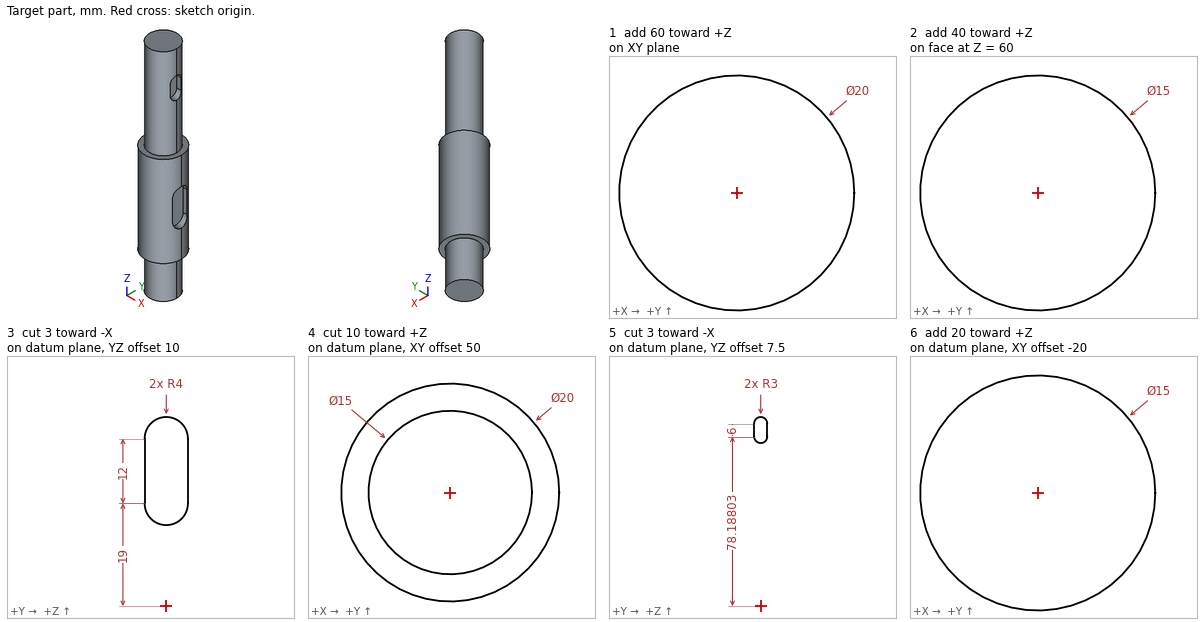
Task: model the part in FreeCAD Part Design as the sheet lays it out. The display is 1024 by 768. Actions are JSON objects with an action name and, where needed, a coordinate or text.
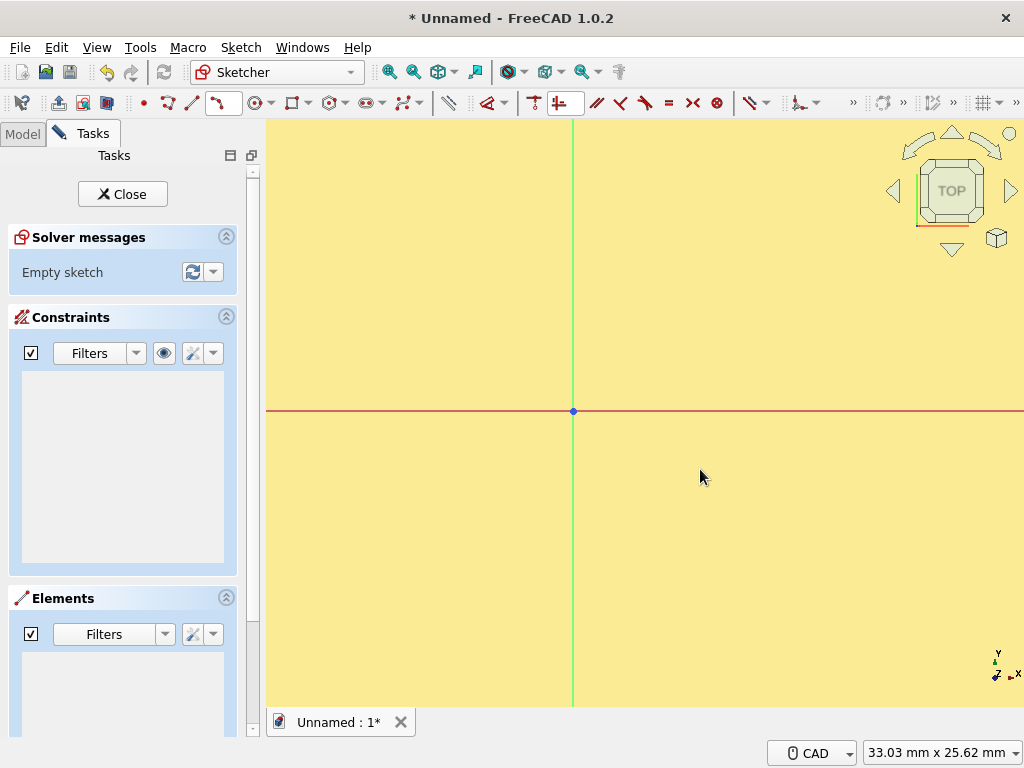
{"action": "left_click", "coordinate": [256, 104]}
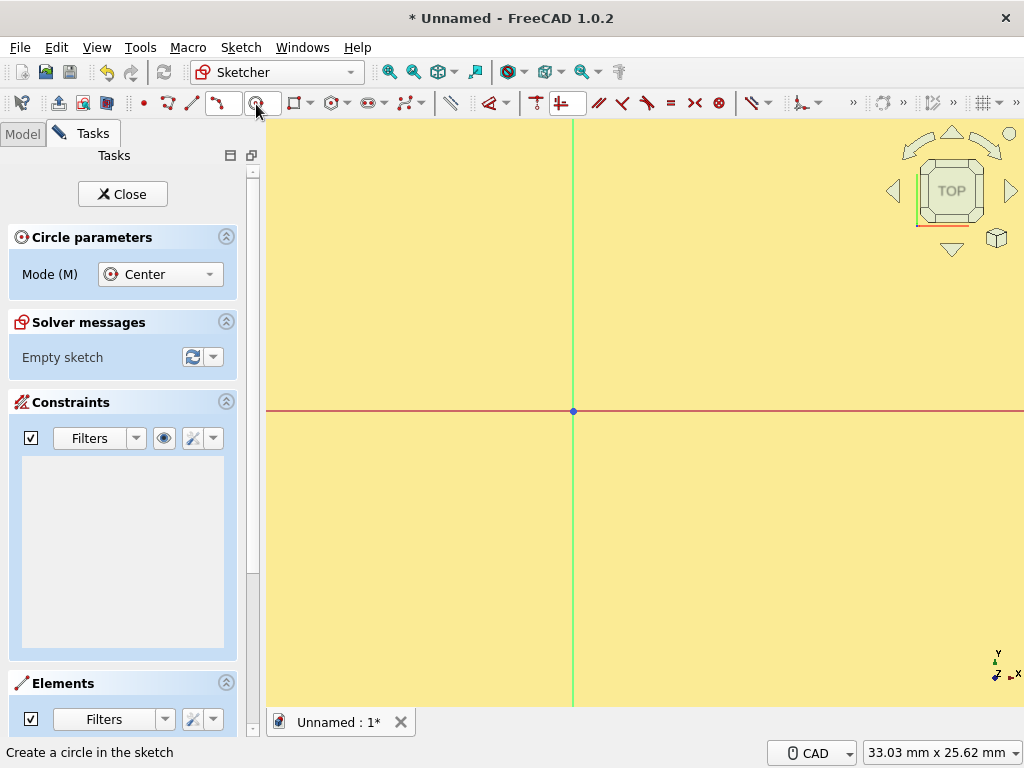
{"action": "left_click", "coordinate": [573, 411]}
{"action": "mouse_move", "coordinate": [695, 290]}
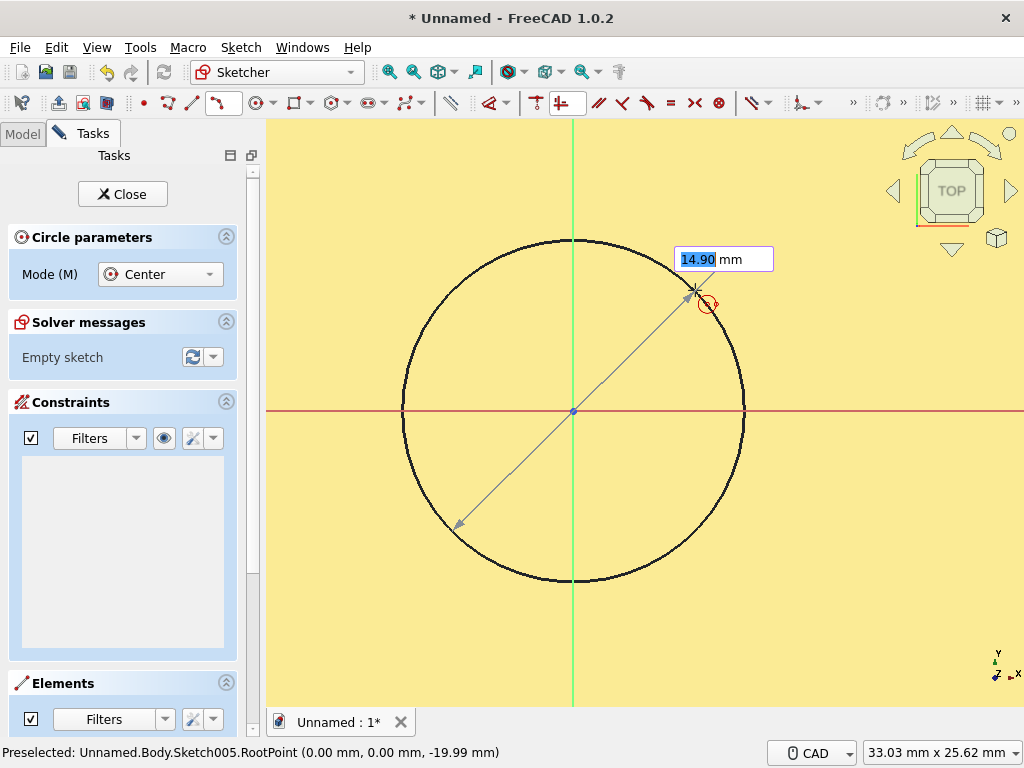
{"action": "type", "text": "15"}
{"action": "key", "text": "Return"}
{"action": "key", "text": "Escape"}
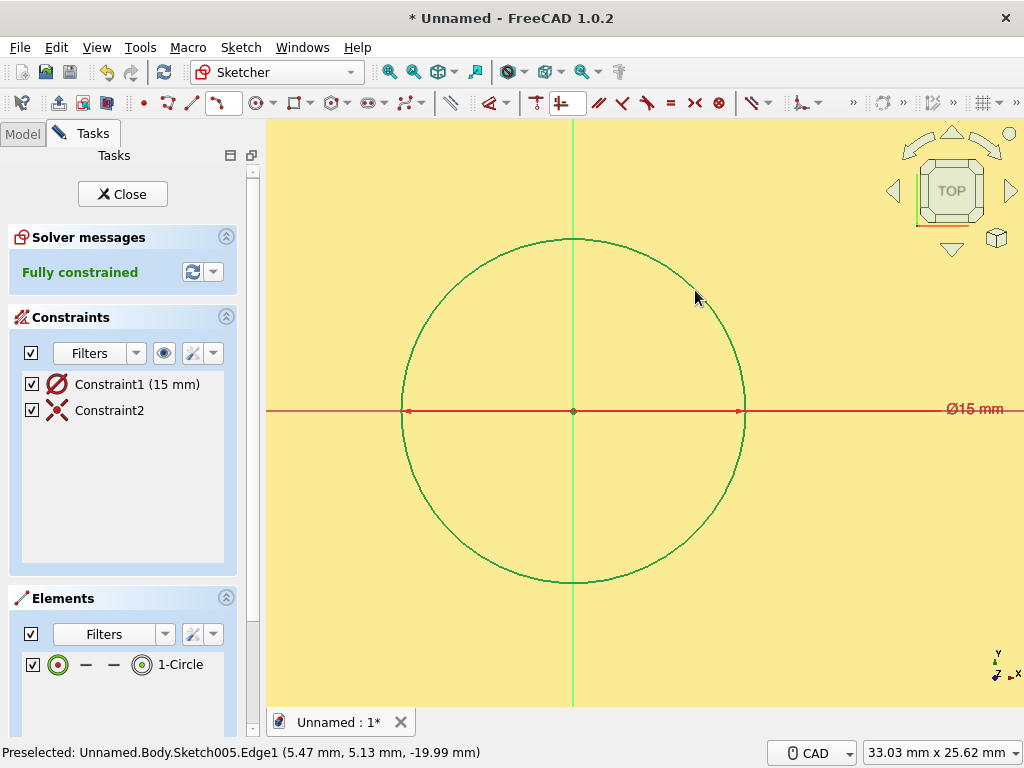
{"action": "left_click", "coordinate": [123, 194]}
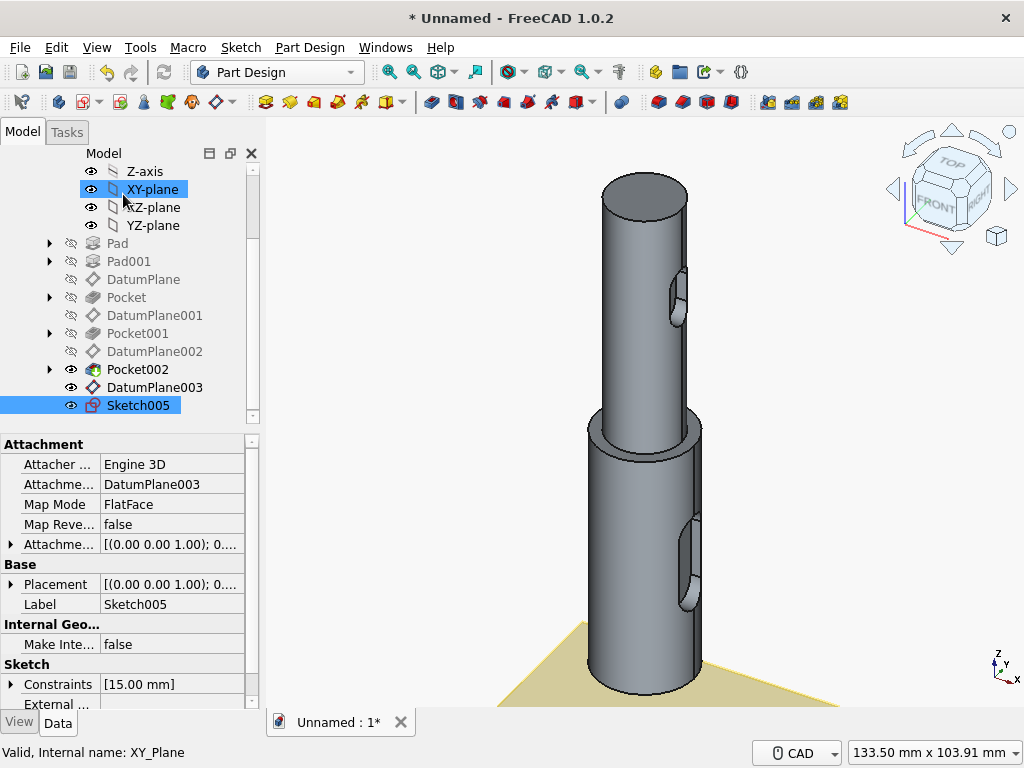
{"action": "left_click", "coordinate": [266, 102]}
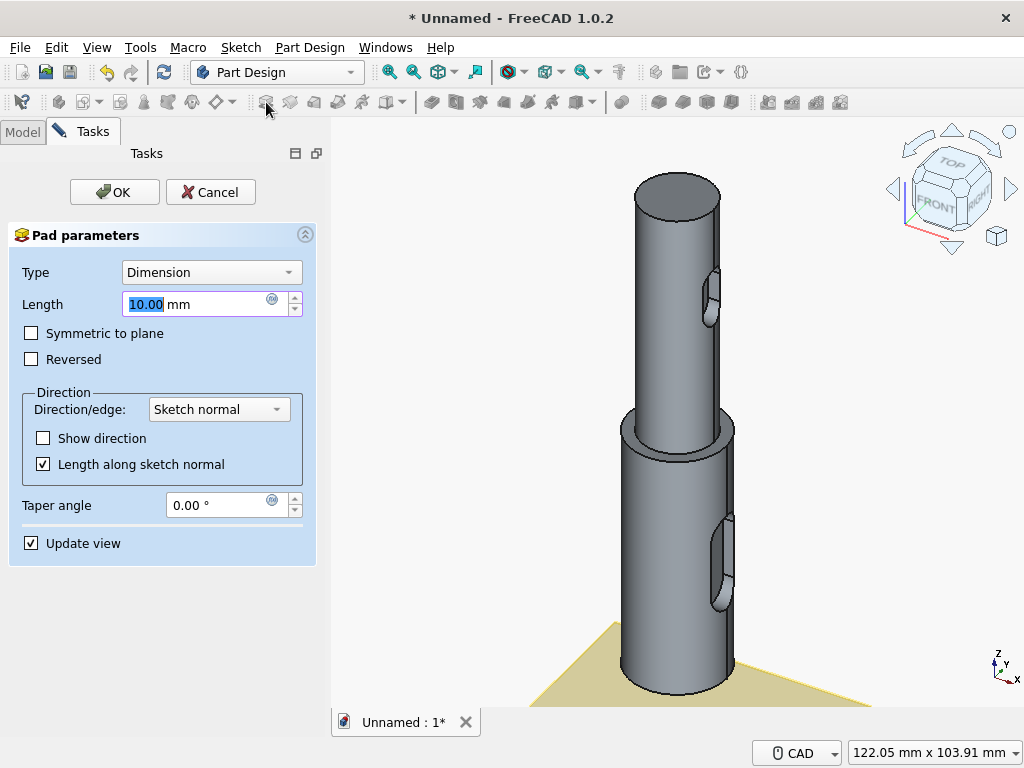
{"action": "type", "text": "20"}
{"action": "key", "text": "Tab"}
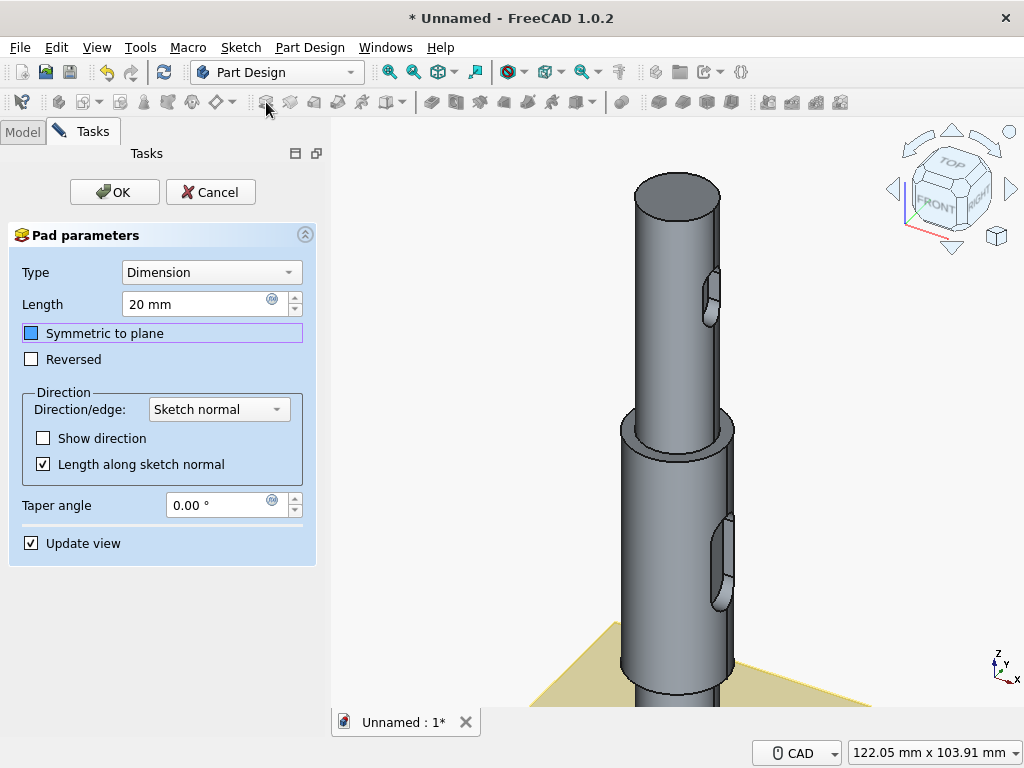
{"action": "left_click", "coordinate": [115, 192]}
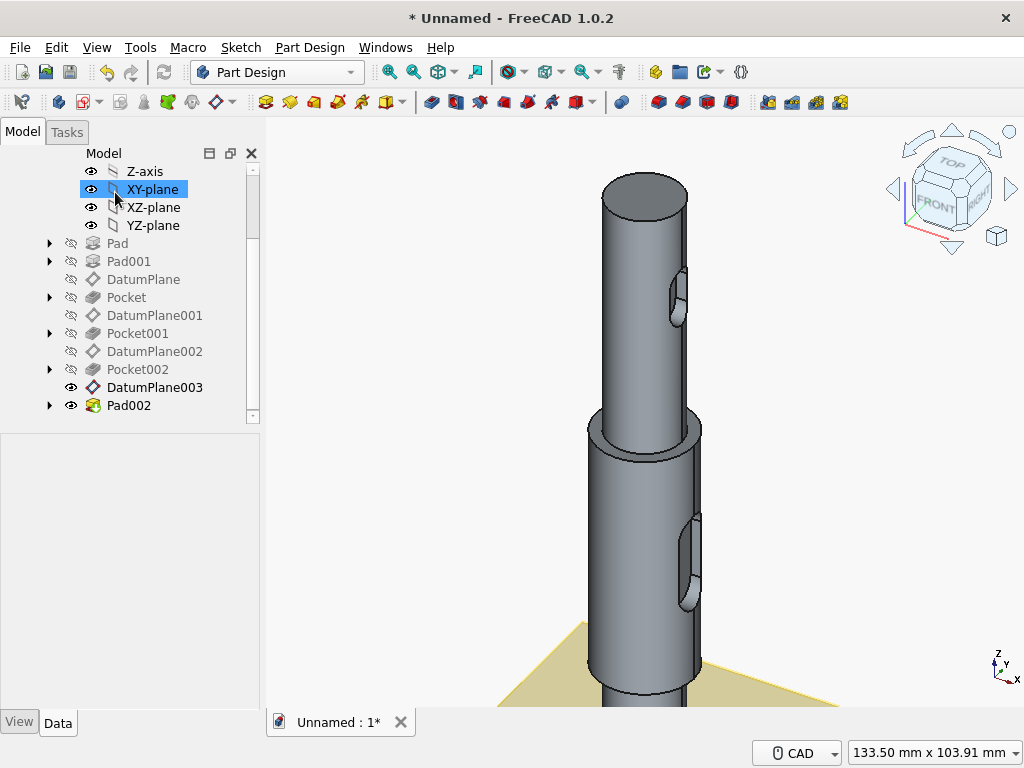
{"action": "left_click", "coordinate": [116, 387]}
{"action": "key", "text": "space"}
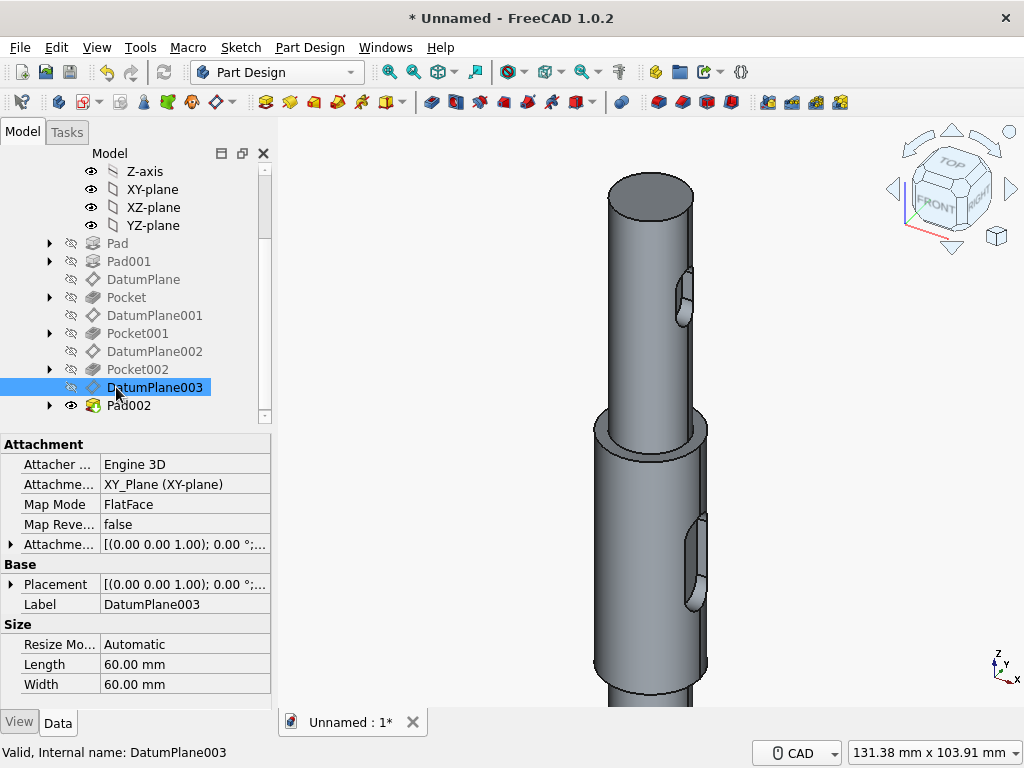
{"action": "key", "text": "0"}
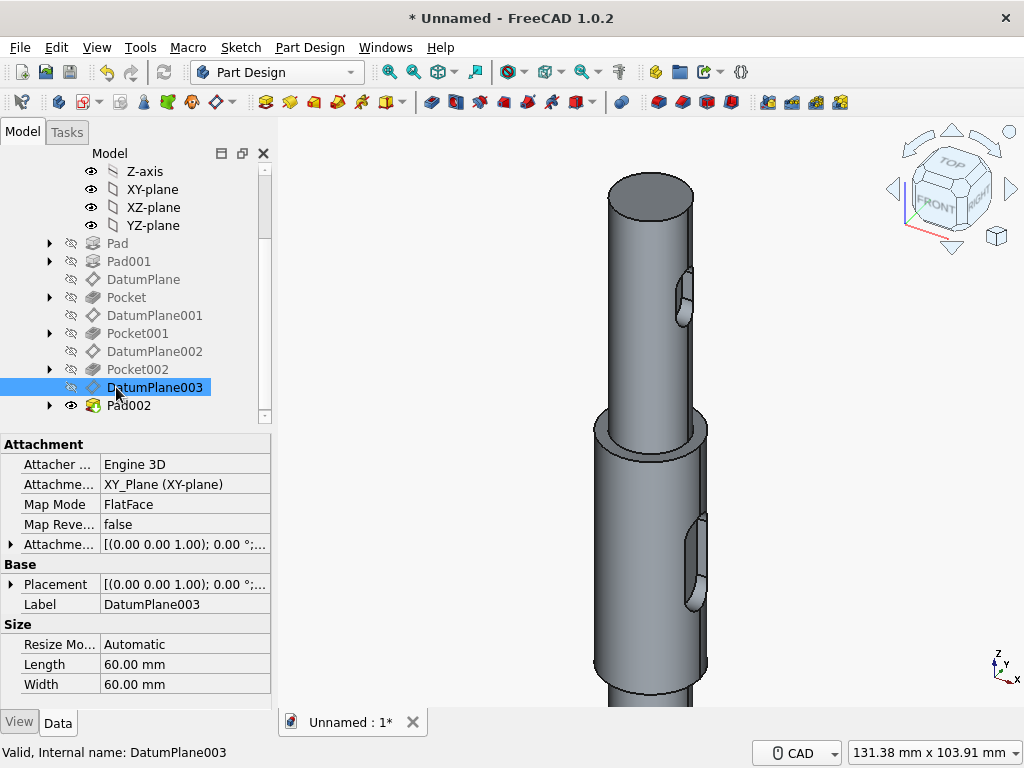
{"action": "left_click", "coordinate": [390, 72]}